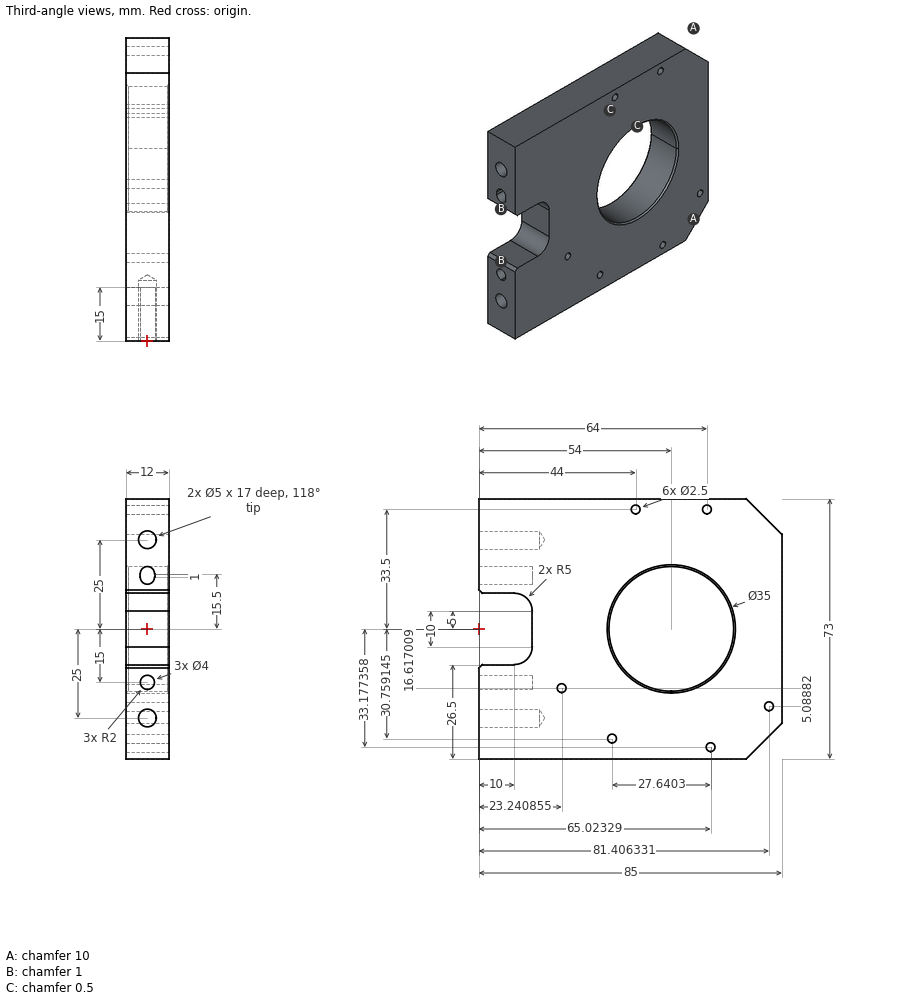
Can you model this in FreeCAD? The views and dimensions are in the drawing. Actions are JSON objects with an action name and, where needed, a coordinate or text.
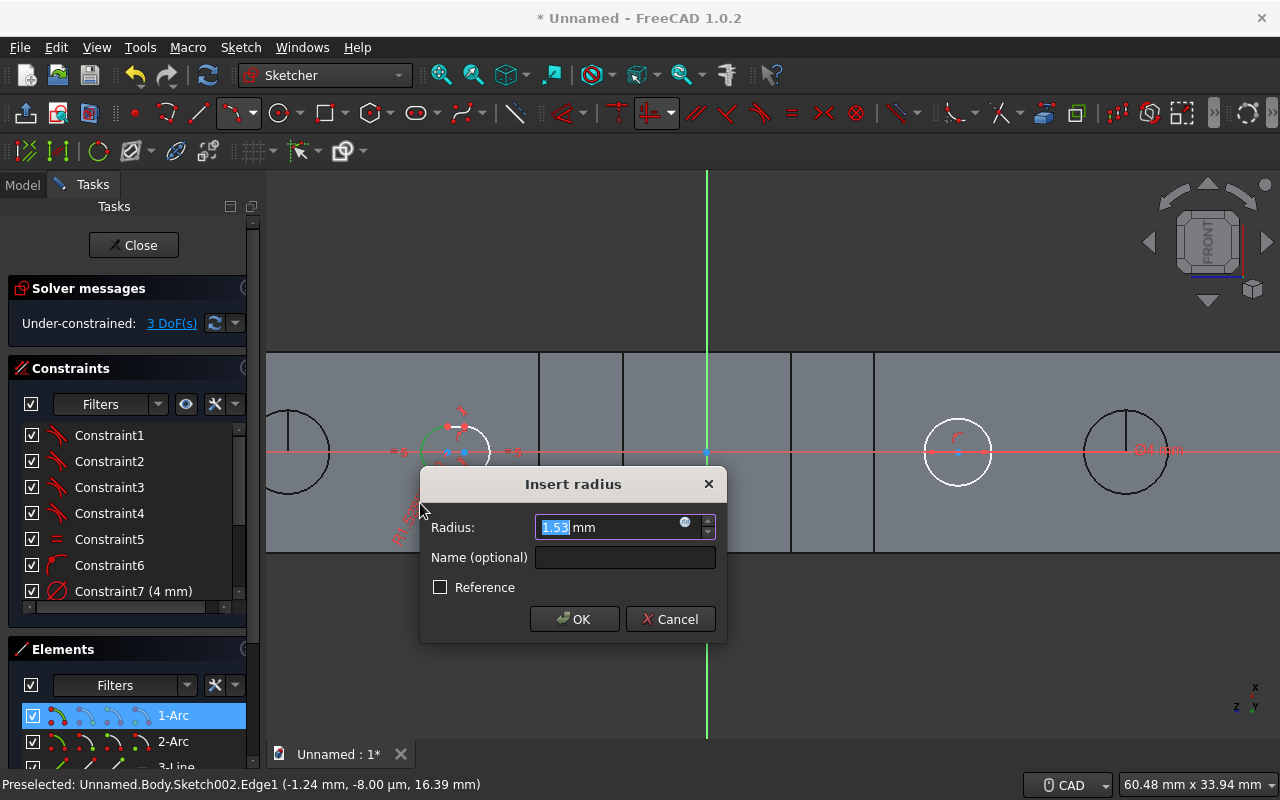
{"action": "type", "text": "2"}
{"action": "key", "text": "Return"}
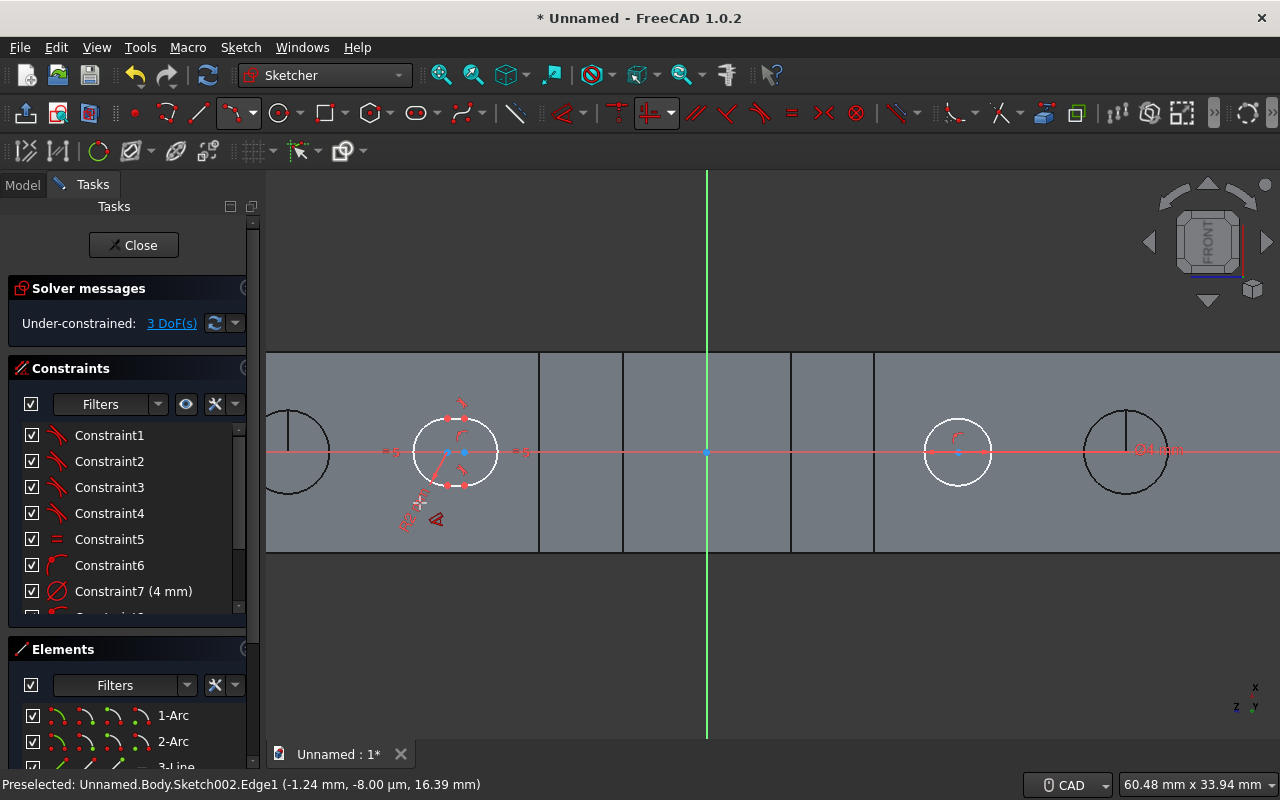
{"action": "scroll", "coordinate": [456, 419], "scroll_direction": "up", "scroll_amount": 5}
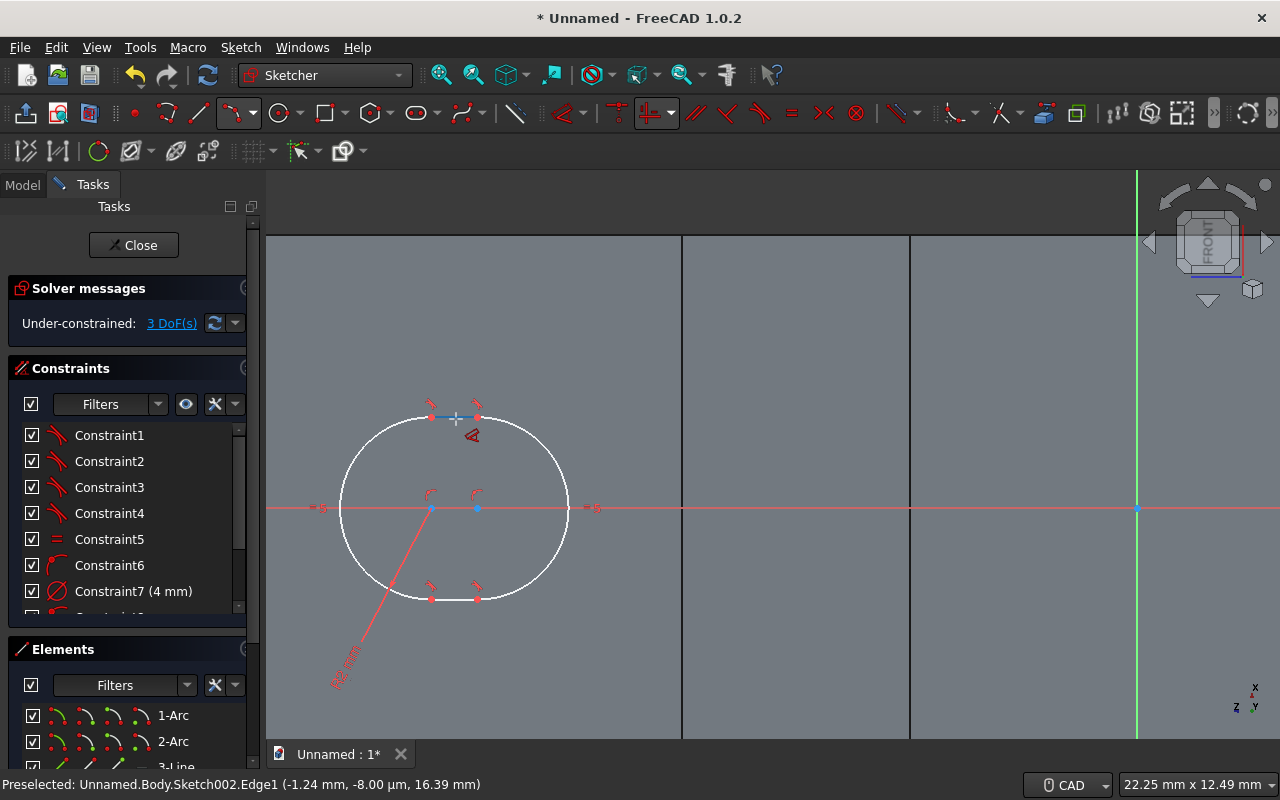
{"action": "left_click", "coordinate": [454, 417]}
{"action": "left_click", "coordinate": [454, 383]}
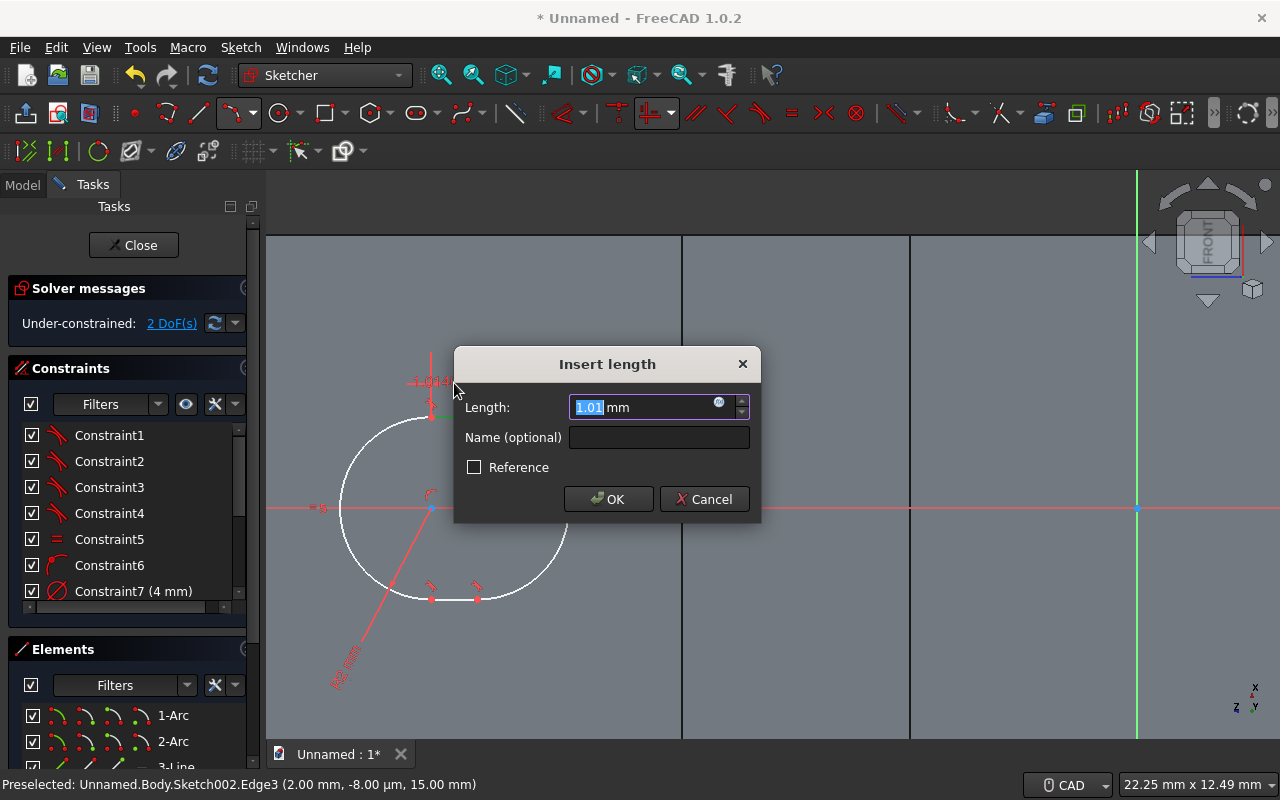
{"action": "type", "text": "1"}
{"action": "key", "text": "Return"}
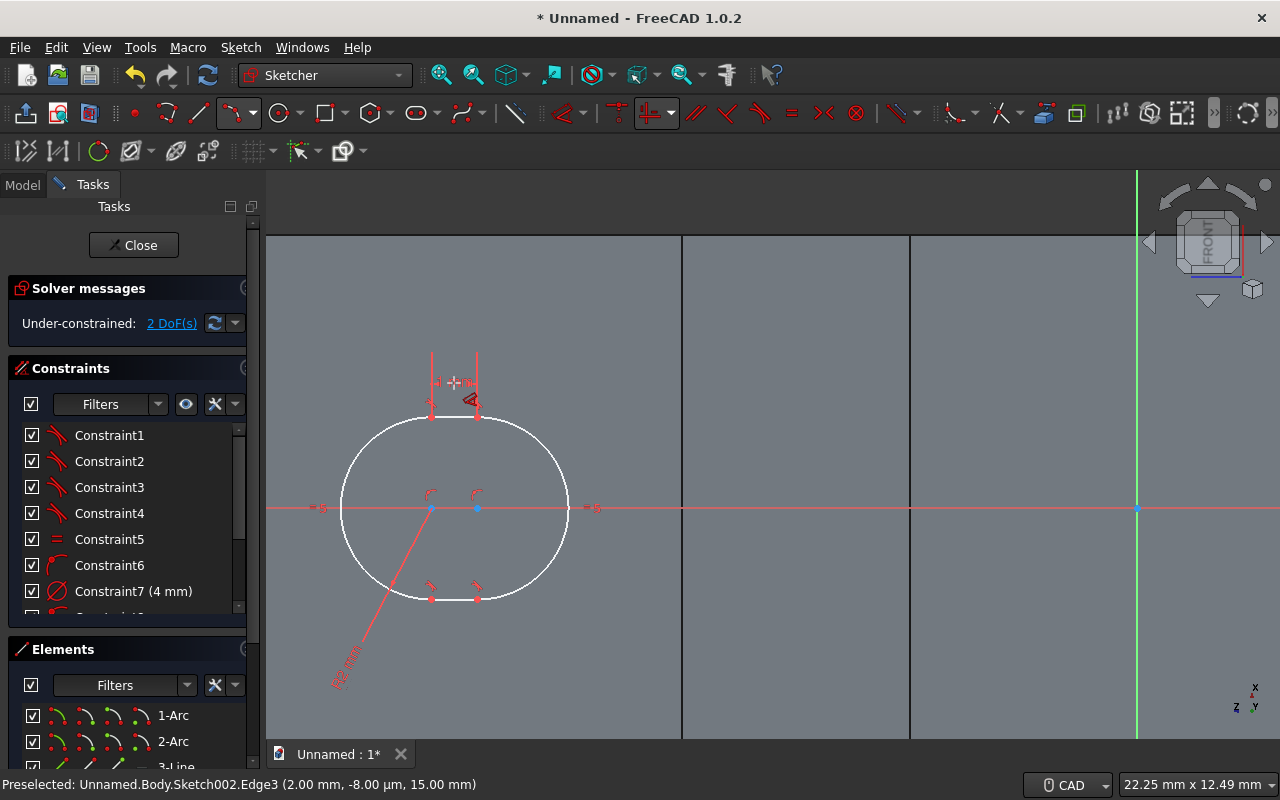
{"action": "scroll", "coordinate": [459, 423], "scroll_direction": "down", "scroll_amount": 5}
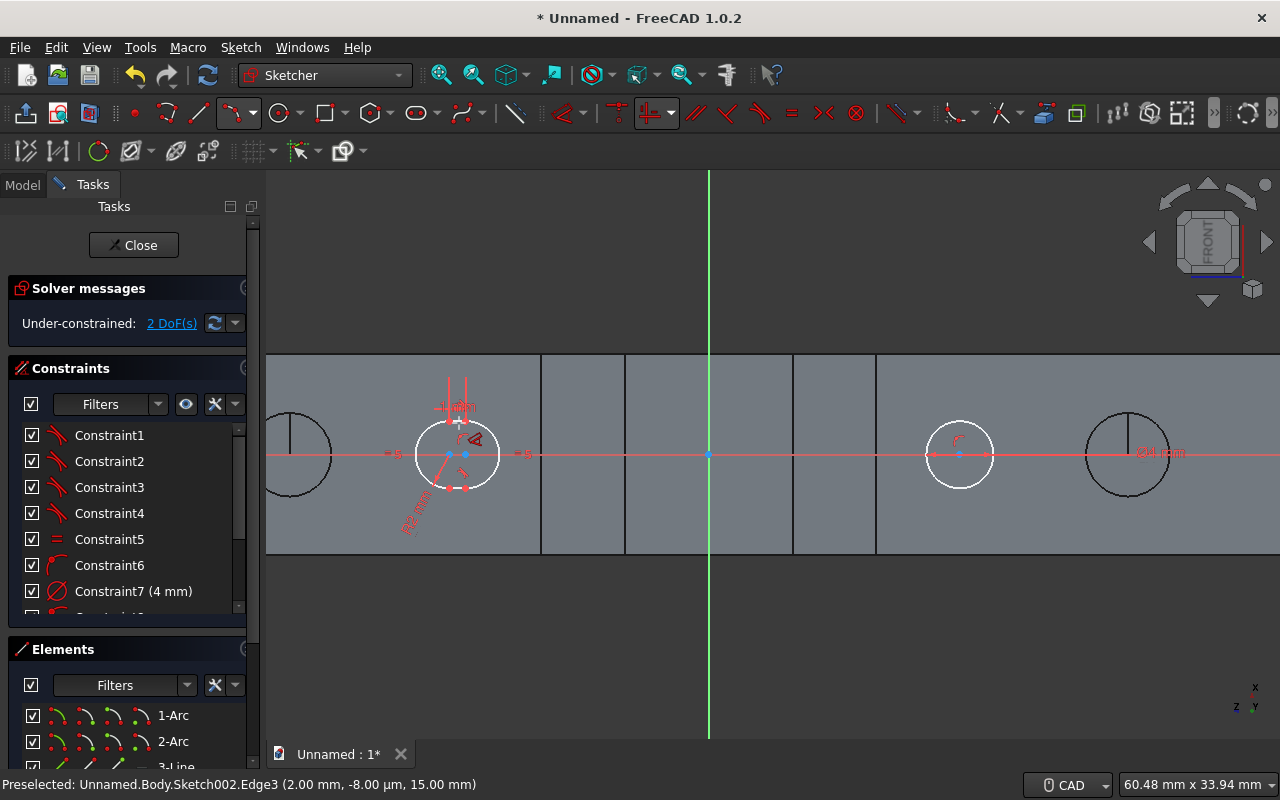
{"action": "left_click", "coordinate": [960, 455]}
{"action": "left_click", "coordinate": [834, 489]}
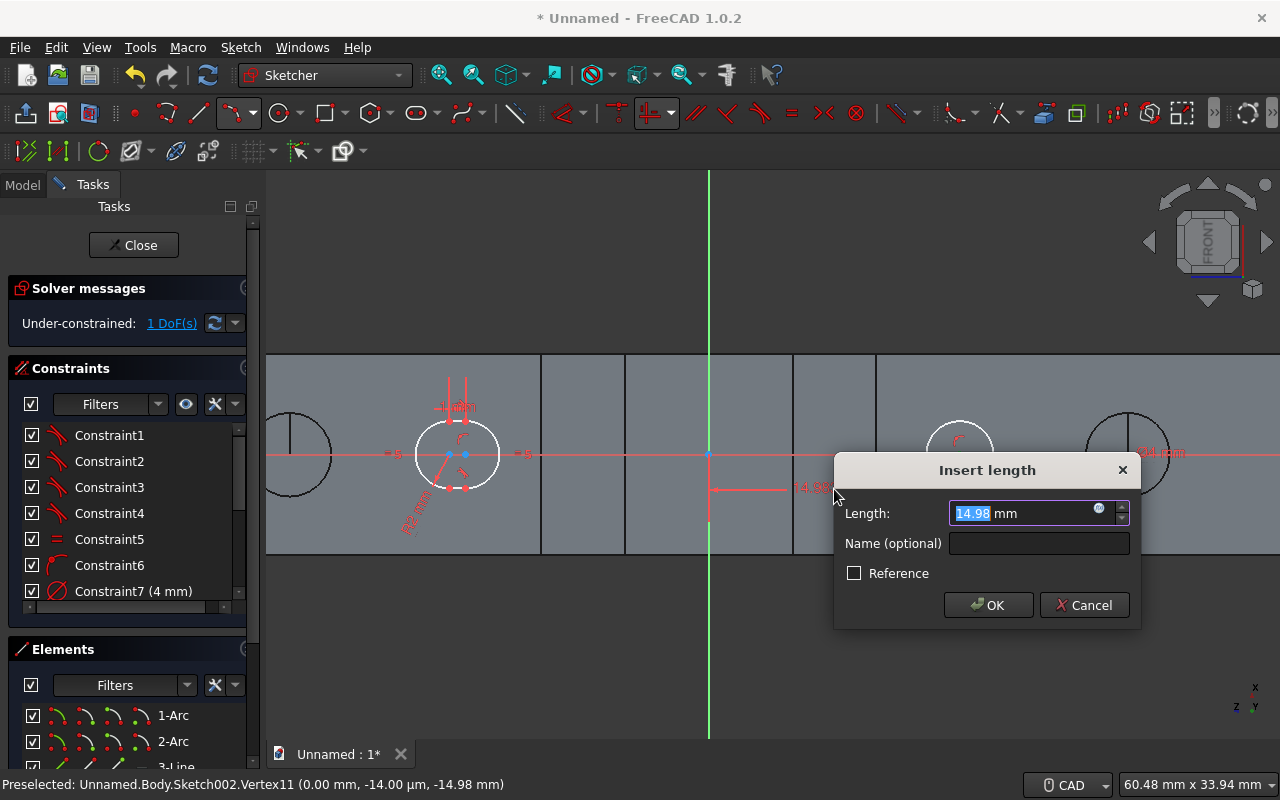
{"action": "type", "text": "15"}
{"action": "key", "text": "Return"}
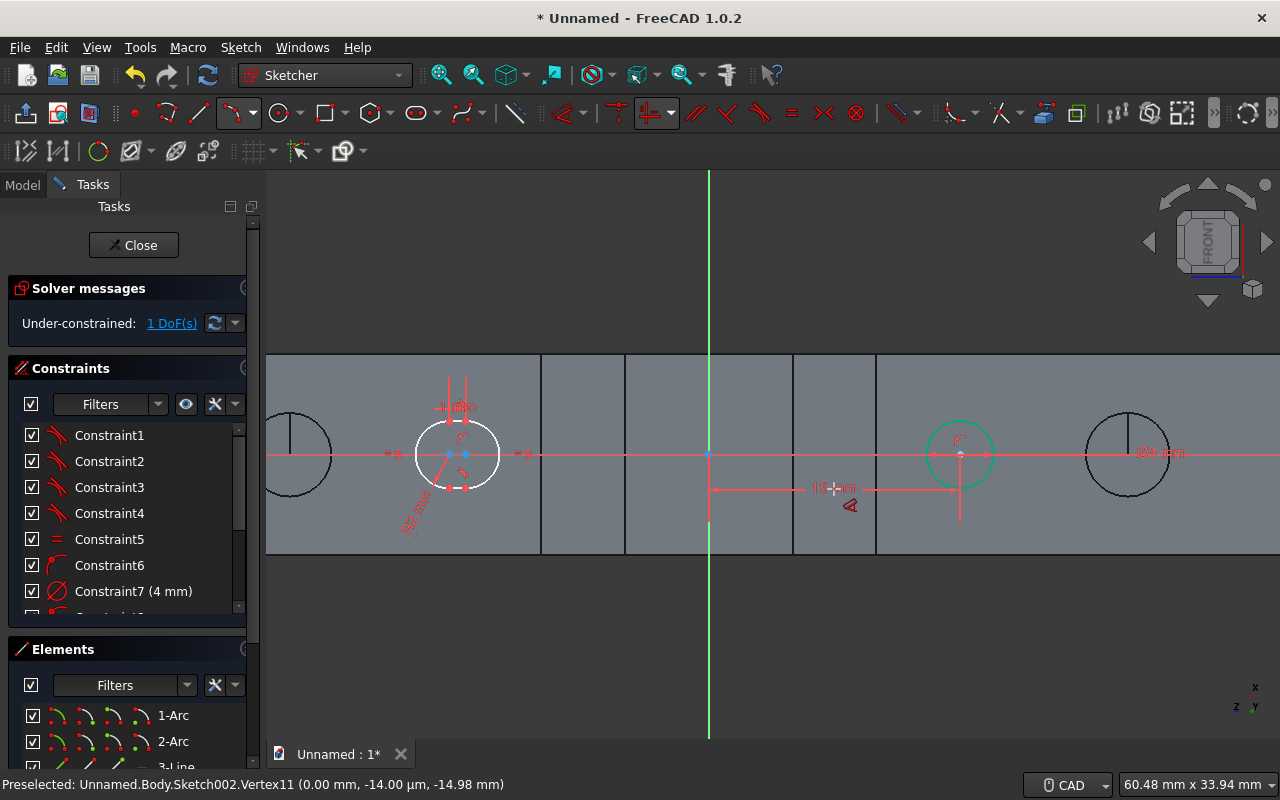
{"action": "left_click", "coordinate": [449, 421]}
{"action": "left_click", "coordinate": [579, 387]}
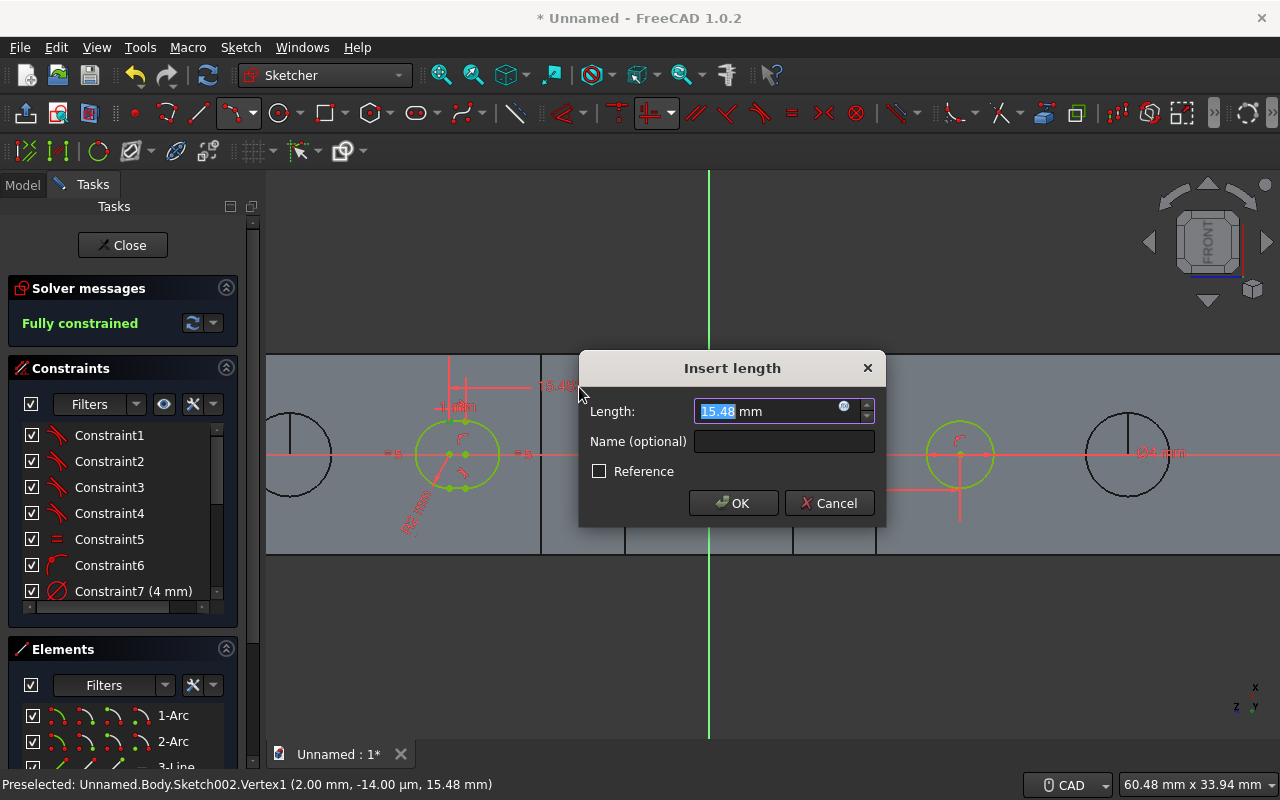
{"action": "type", "text": "15.5"}
{"action": "key", "text": "Return"}
{"action": "key", "text": "Escape"}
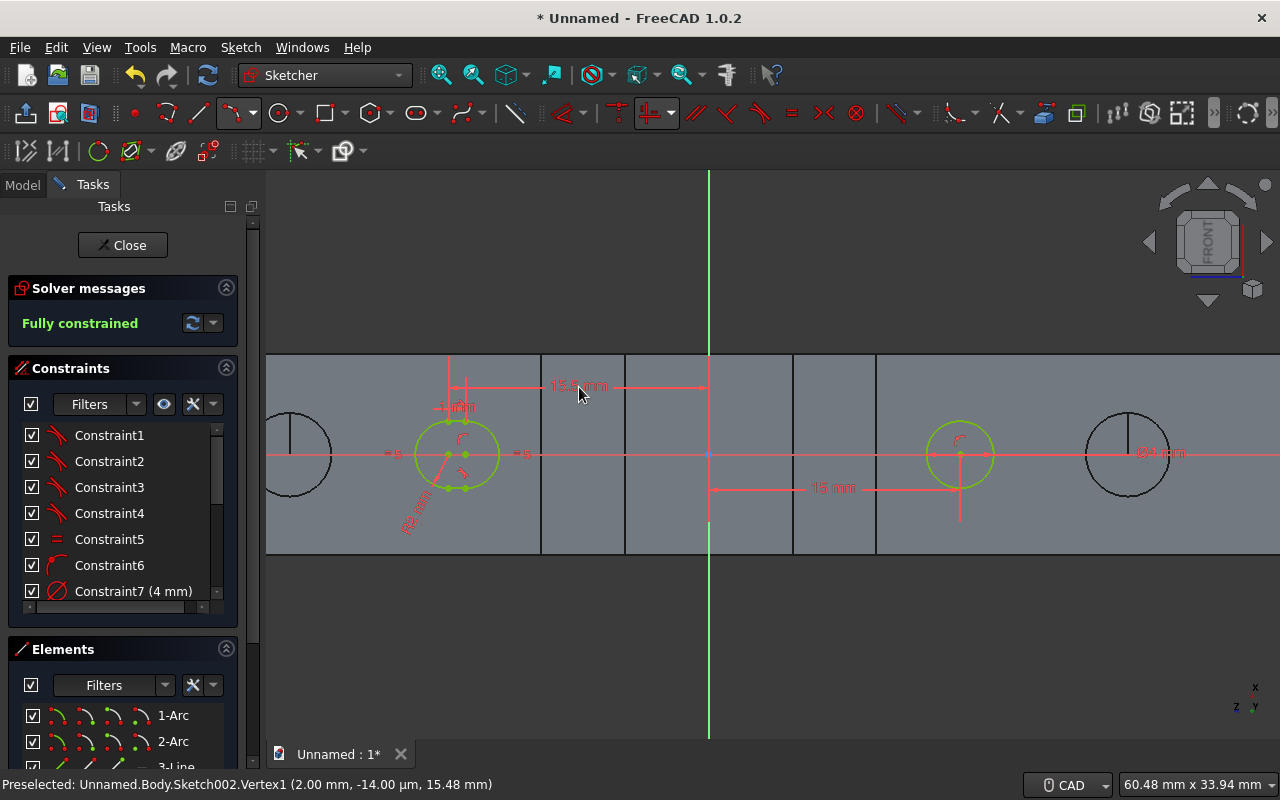
{"action": "left_click", "coordinate": [123, 245]}